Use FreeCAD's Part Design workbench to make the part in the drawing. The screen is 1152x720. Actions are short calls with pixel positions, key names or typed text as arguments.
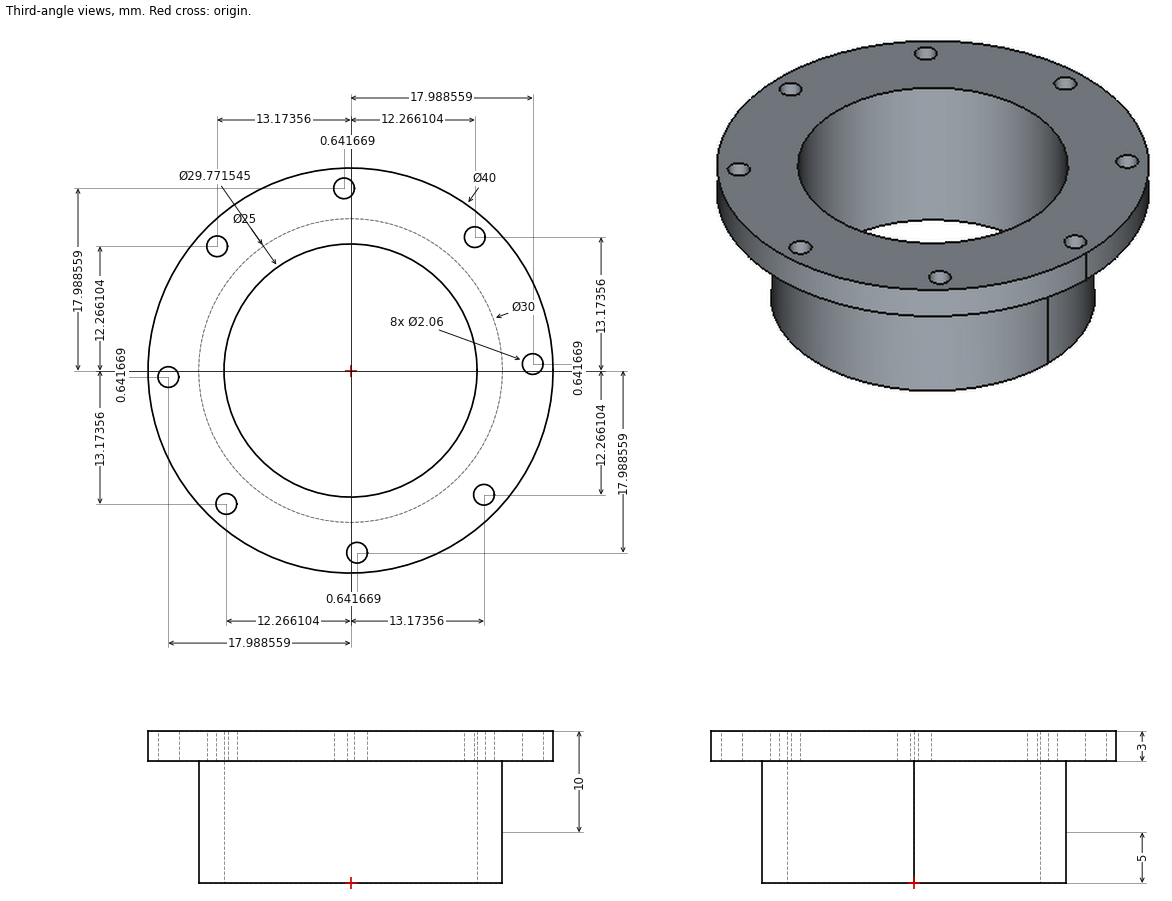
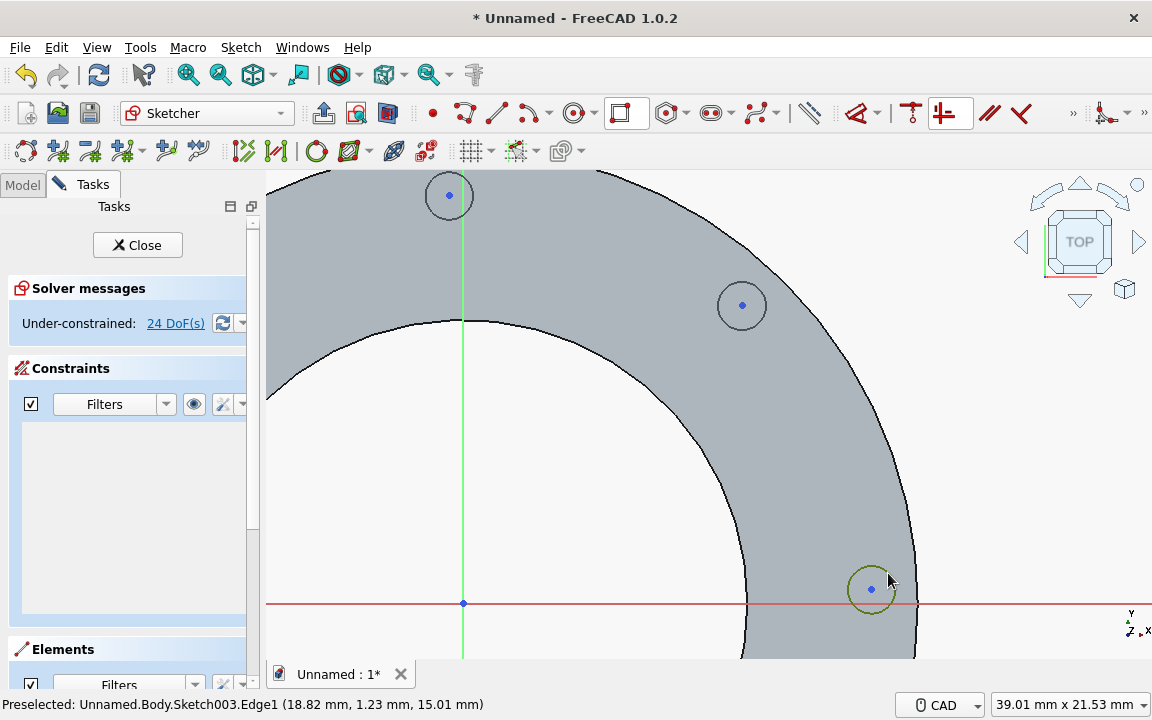
scroll(744, 304, down, 5)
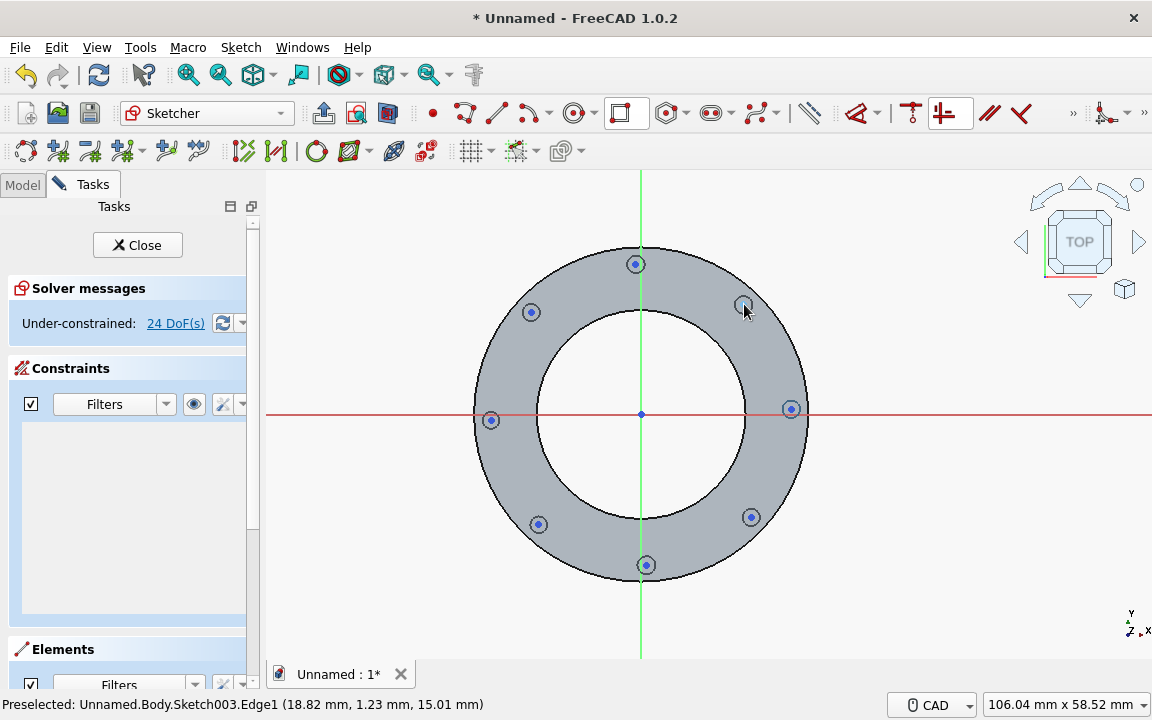
scroll(757, 511, up, 3)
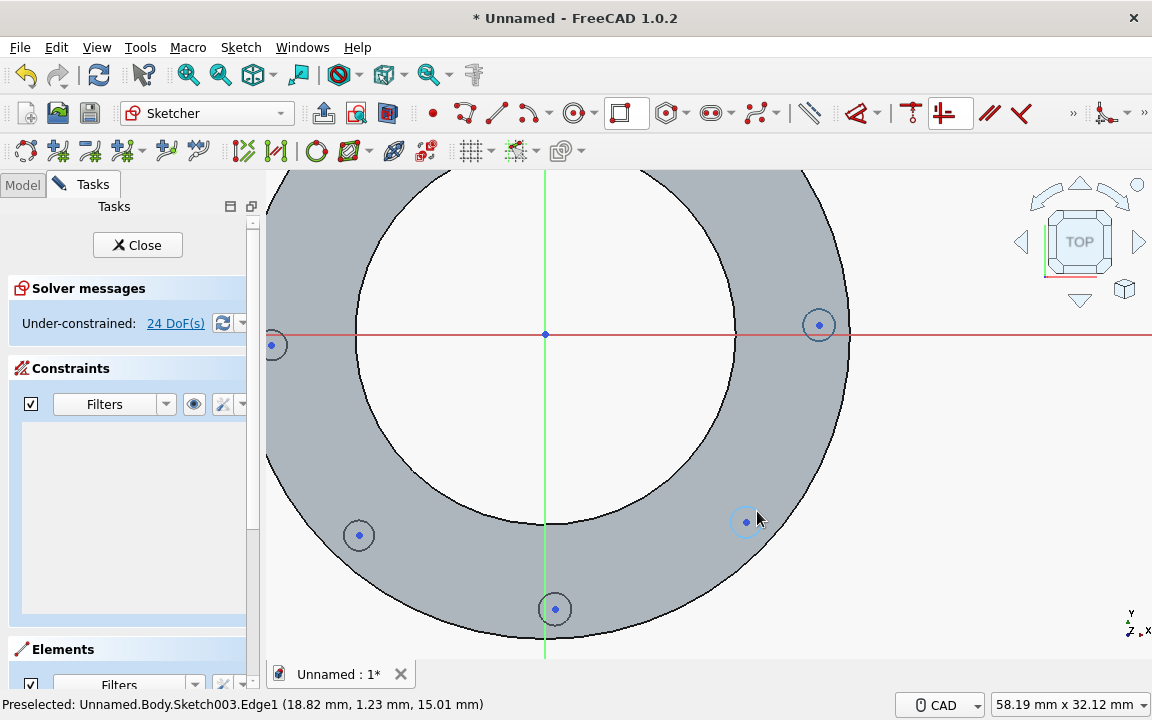
click(757, 511)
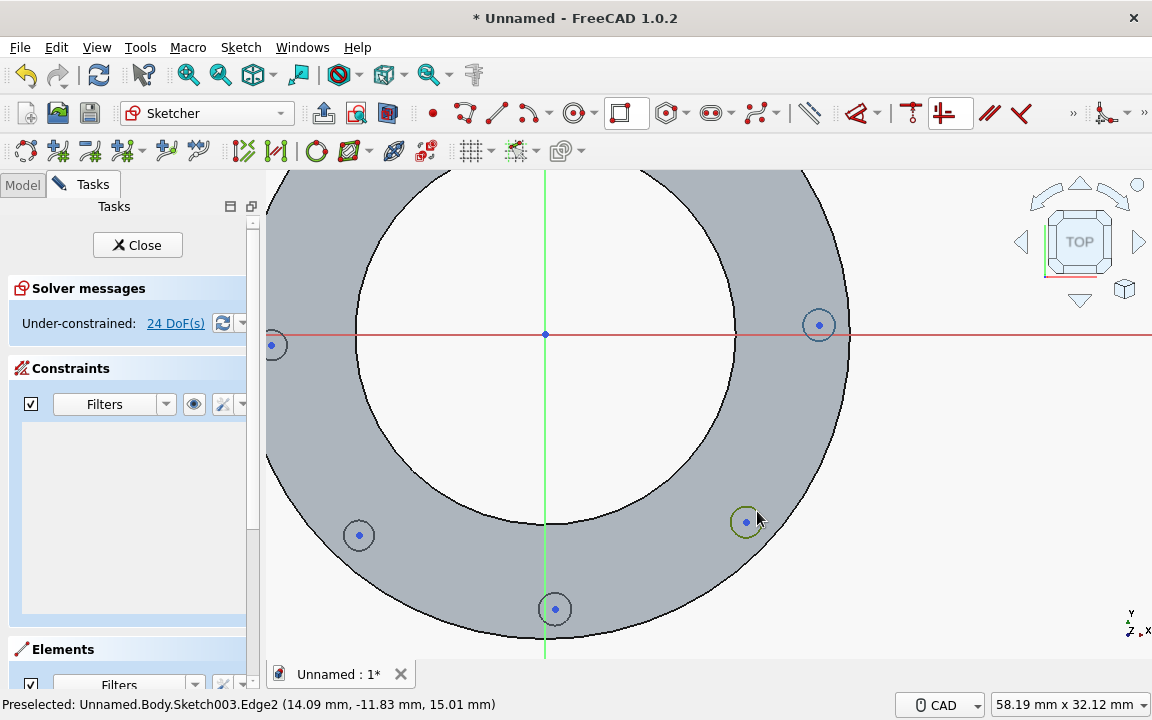
click(567, 598)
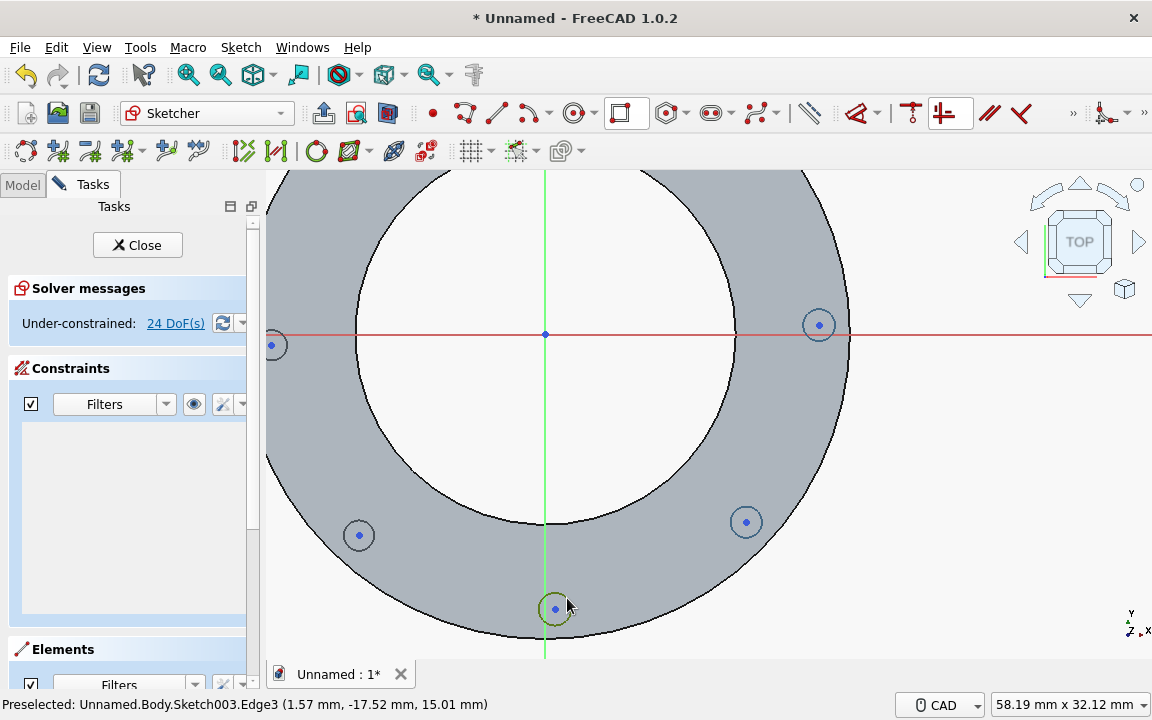
click(370, 525)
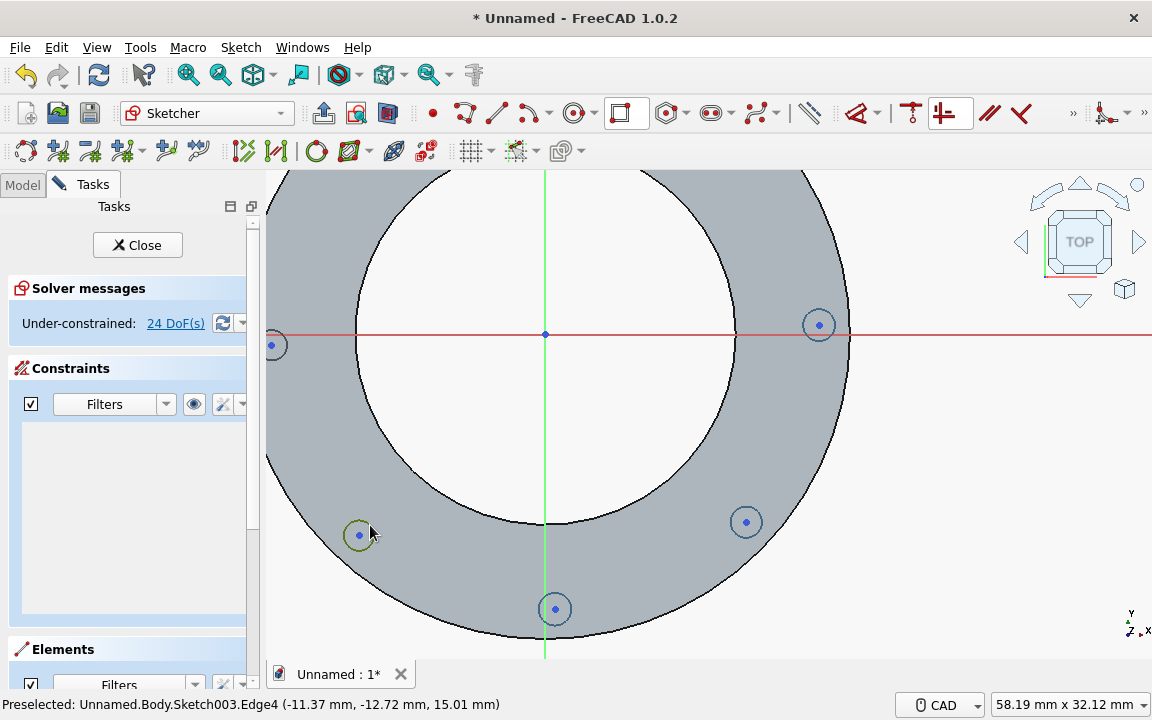
scroll(756, 512, down, 3)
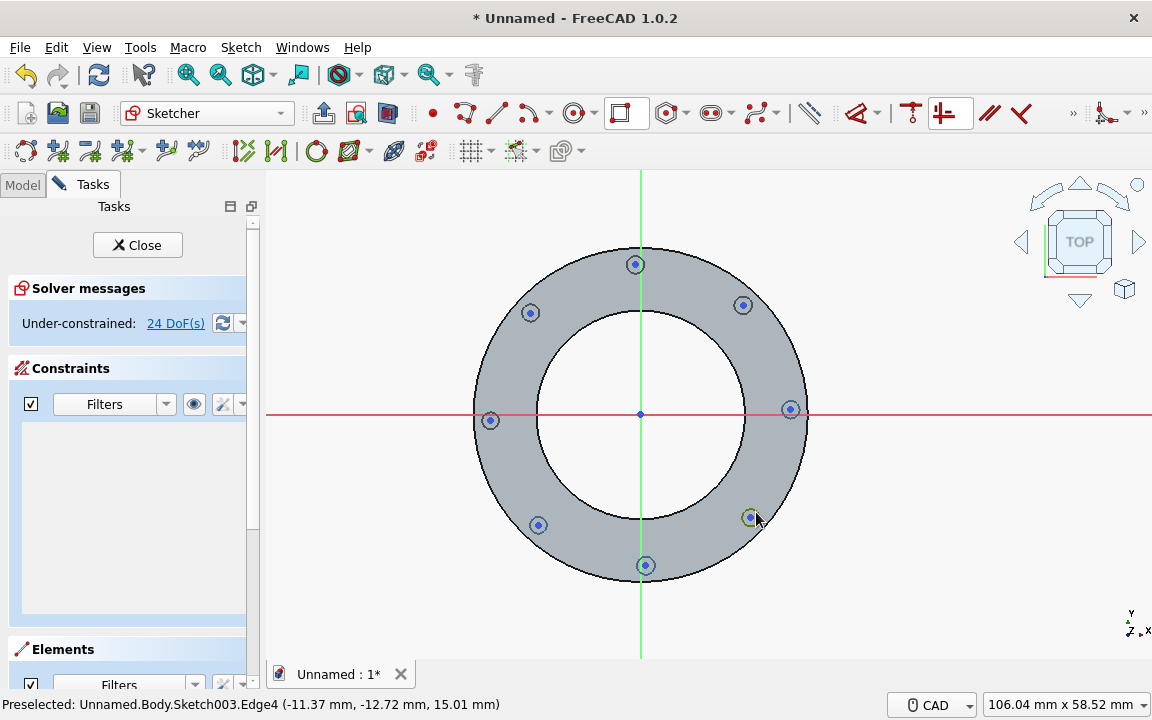
scroll(496, 415, up, 3)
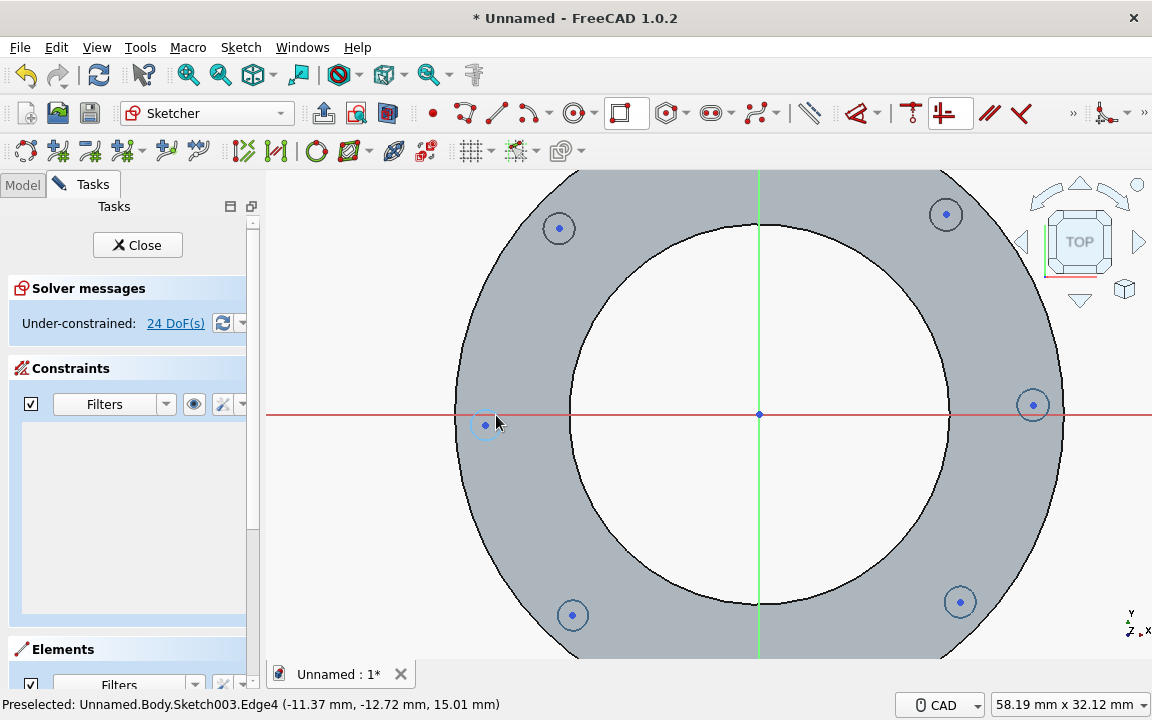
click(497, 414)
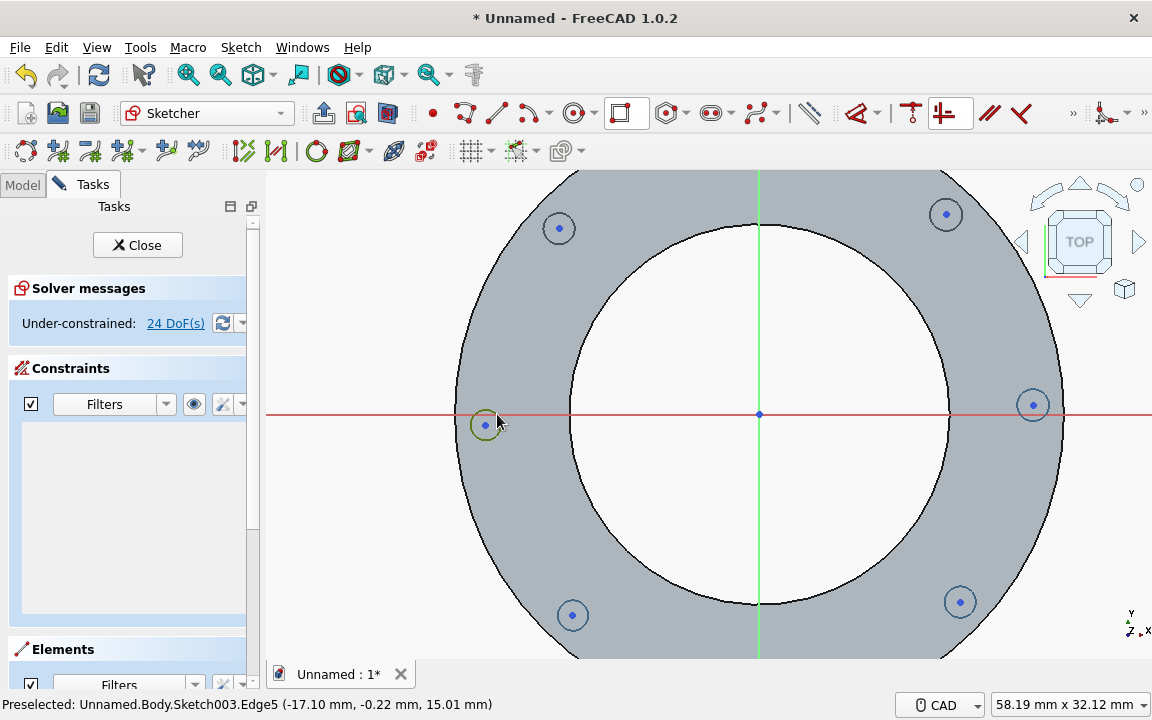
click(570, 218)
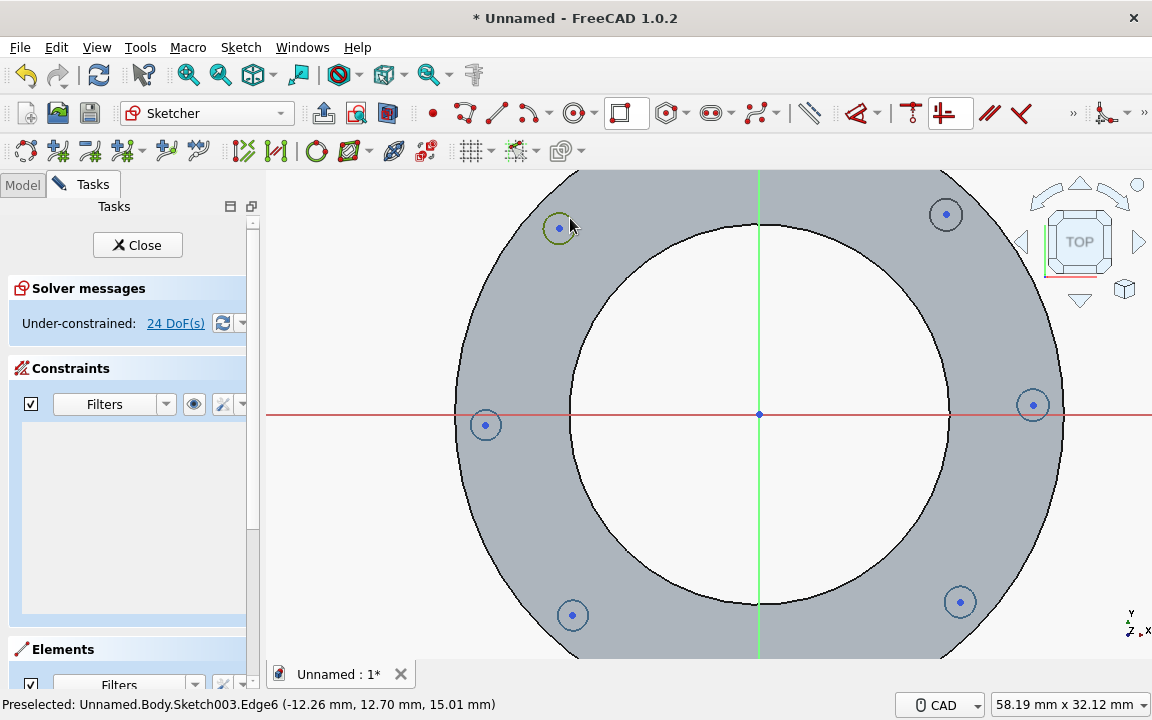
scroll(496, 414, down, 3)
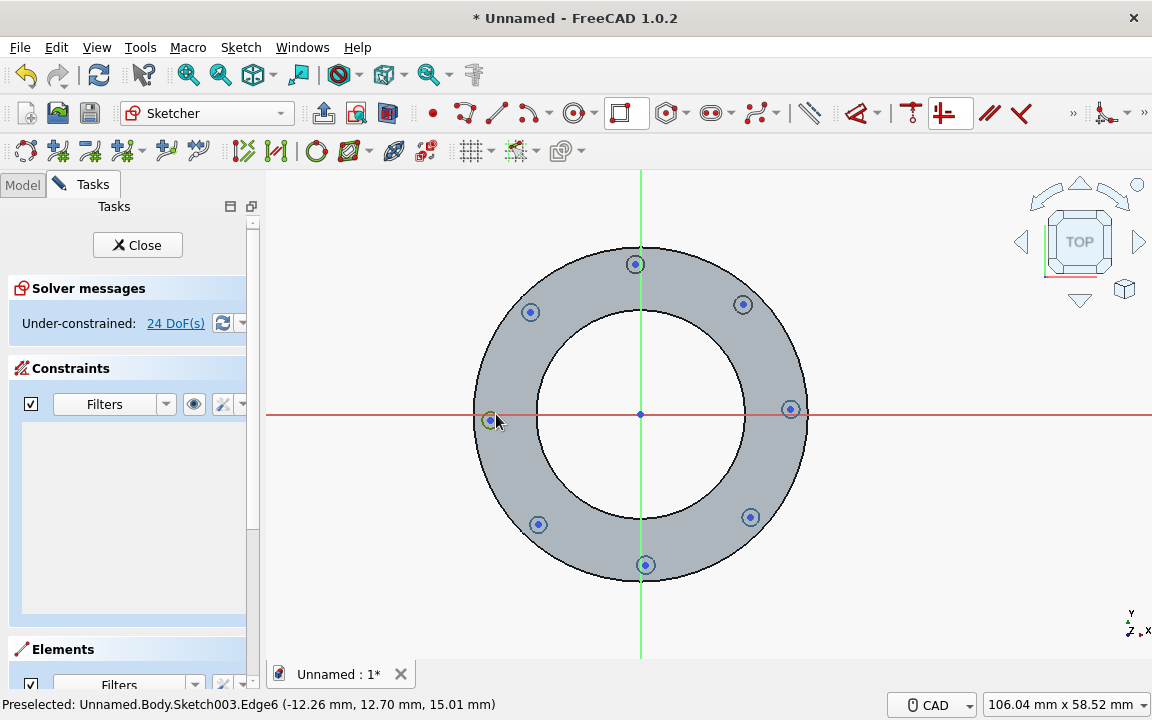
scroll(642, 258, up, 3)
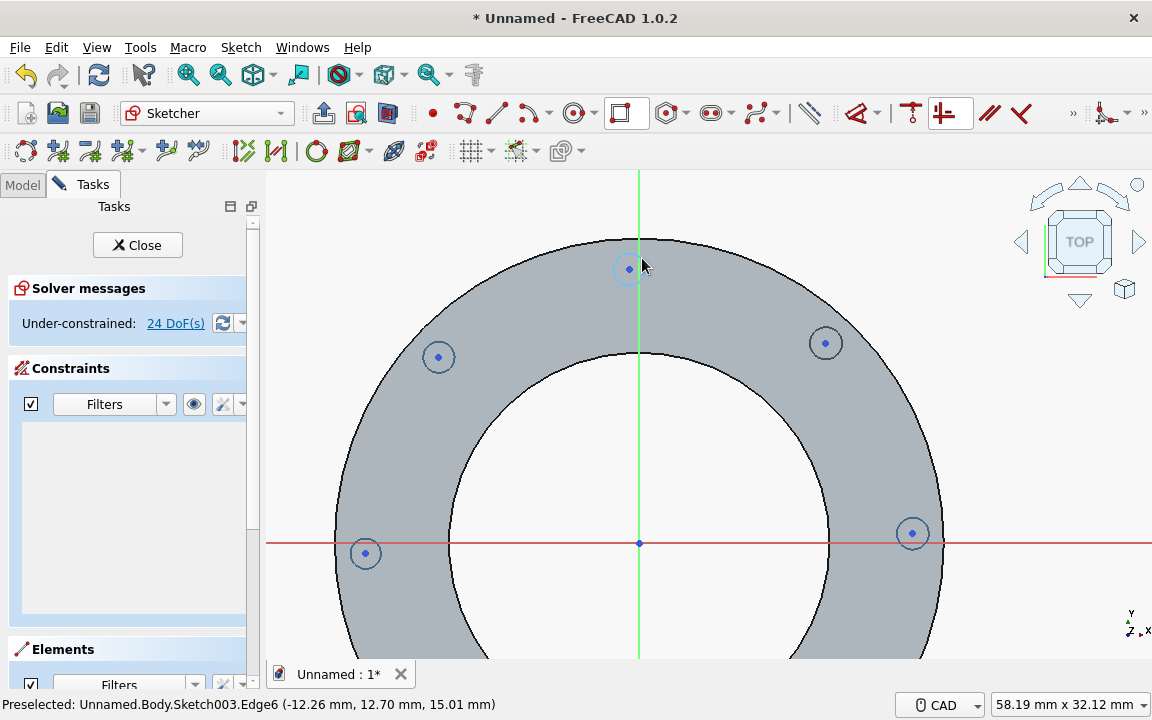
click(641, 258)